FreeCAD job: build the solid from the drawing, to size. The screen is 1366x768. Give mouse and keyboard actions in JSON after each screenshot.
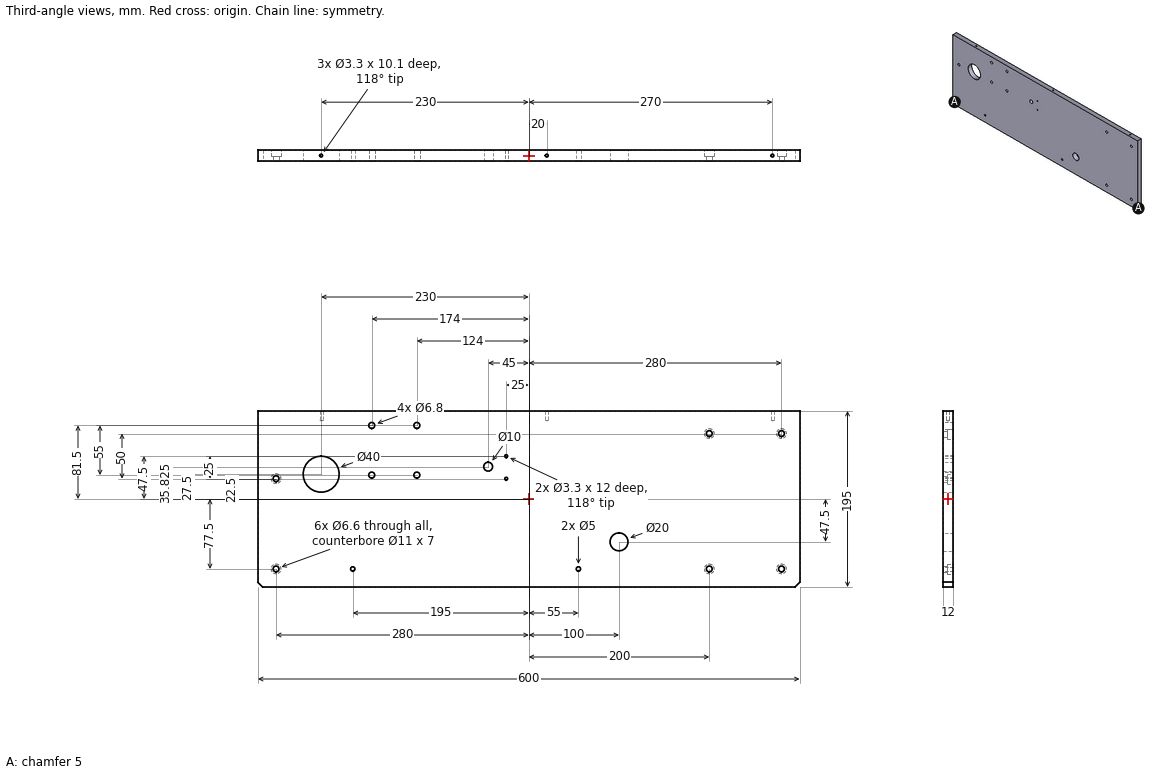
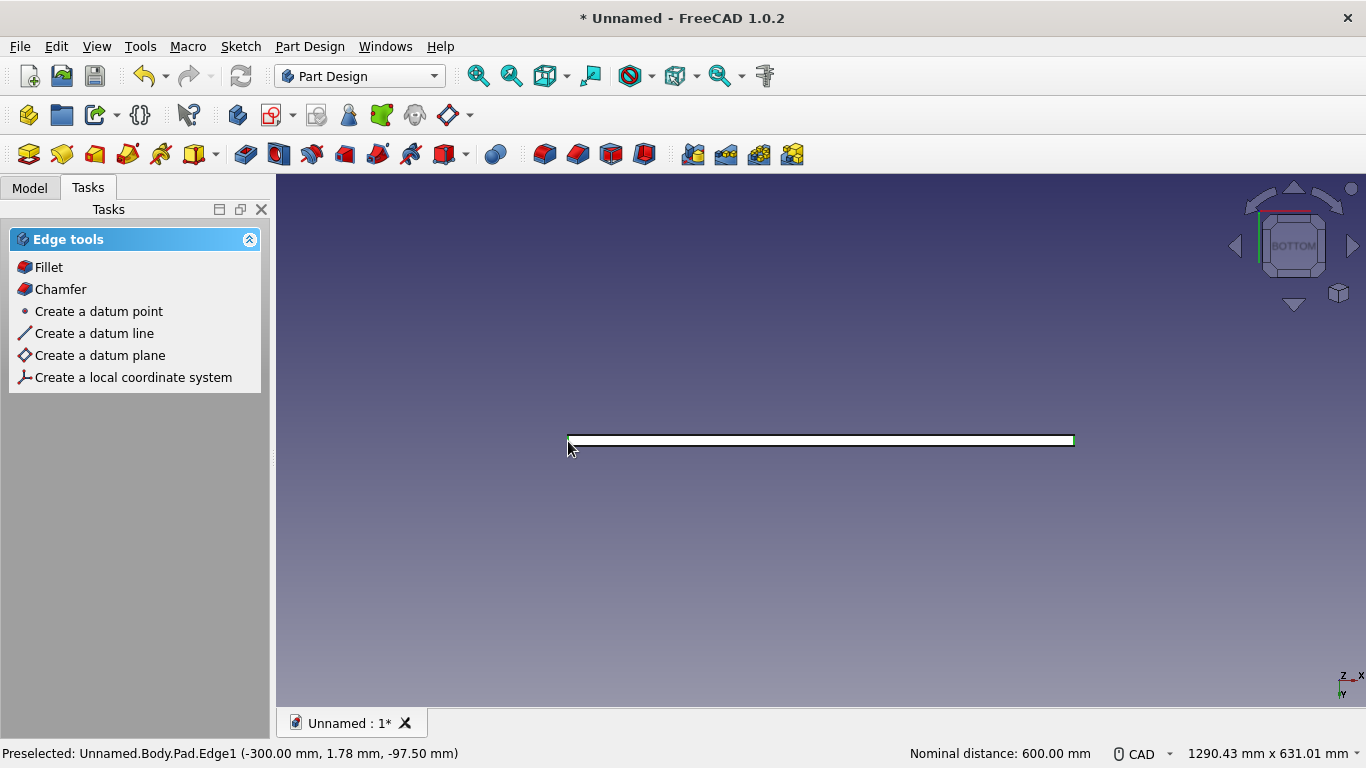
{"action": "left_click", "coordinate": [578, 154]}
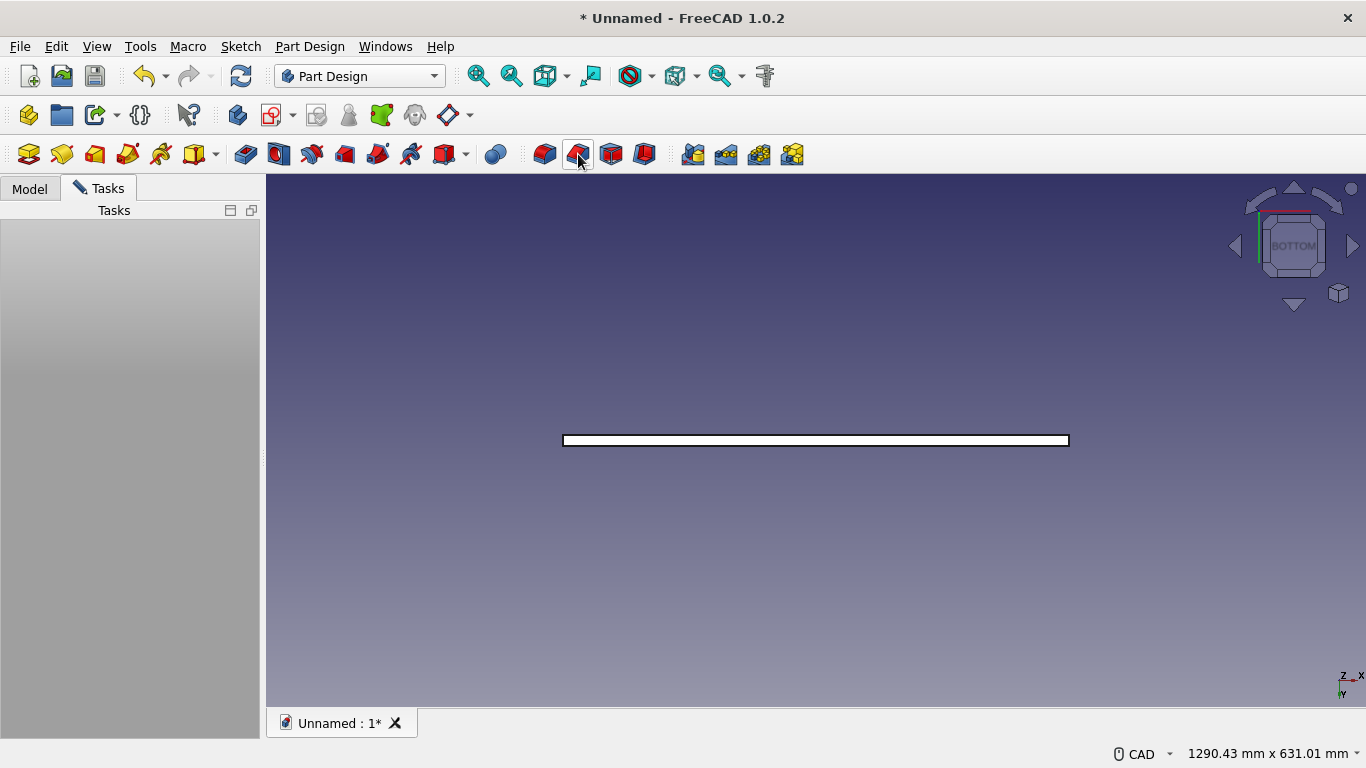
{"action": "type", "text": "5"}
{"action": "key", "text": "Tab"}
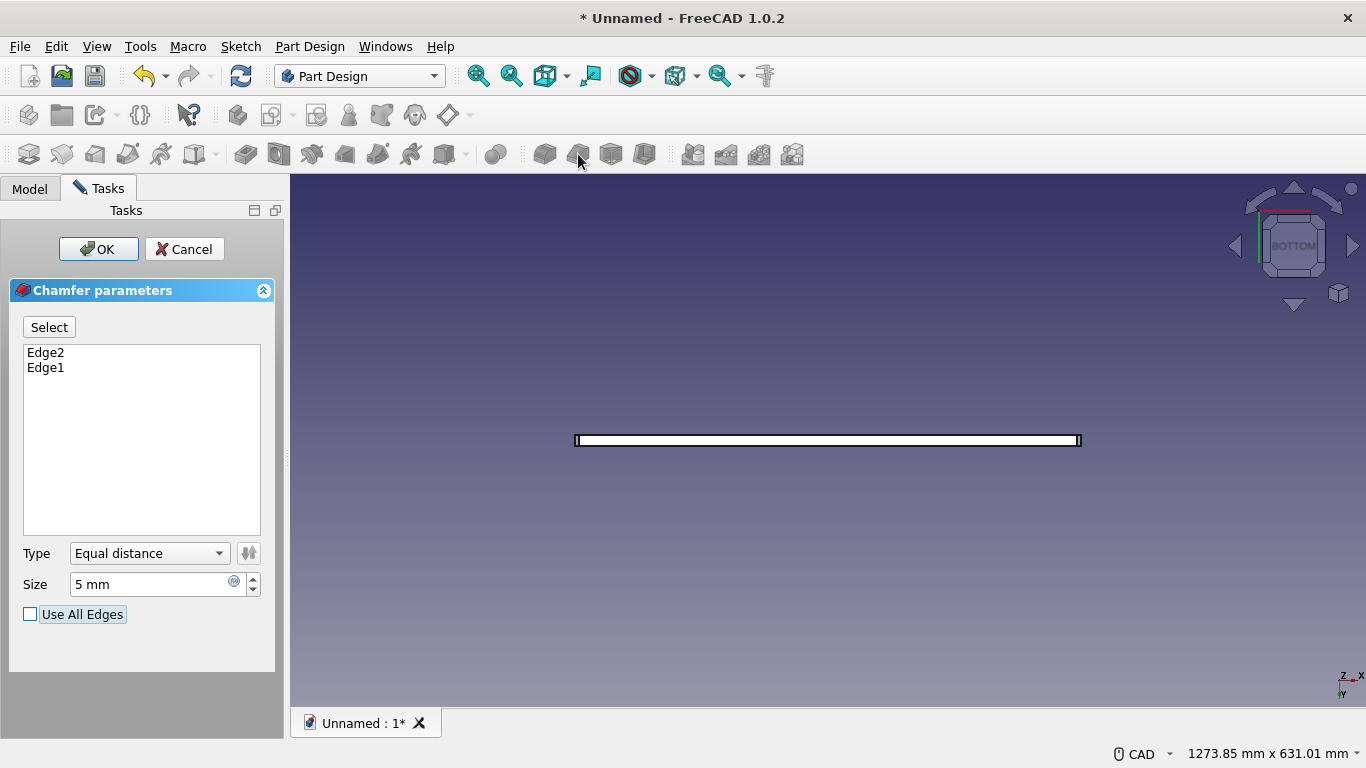
{"action": "left_click", "coordinate": [99, 249]}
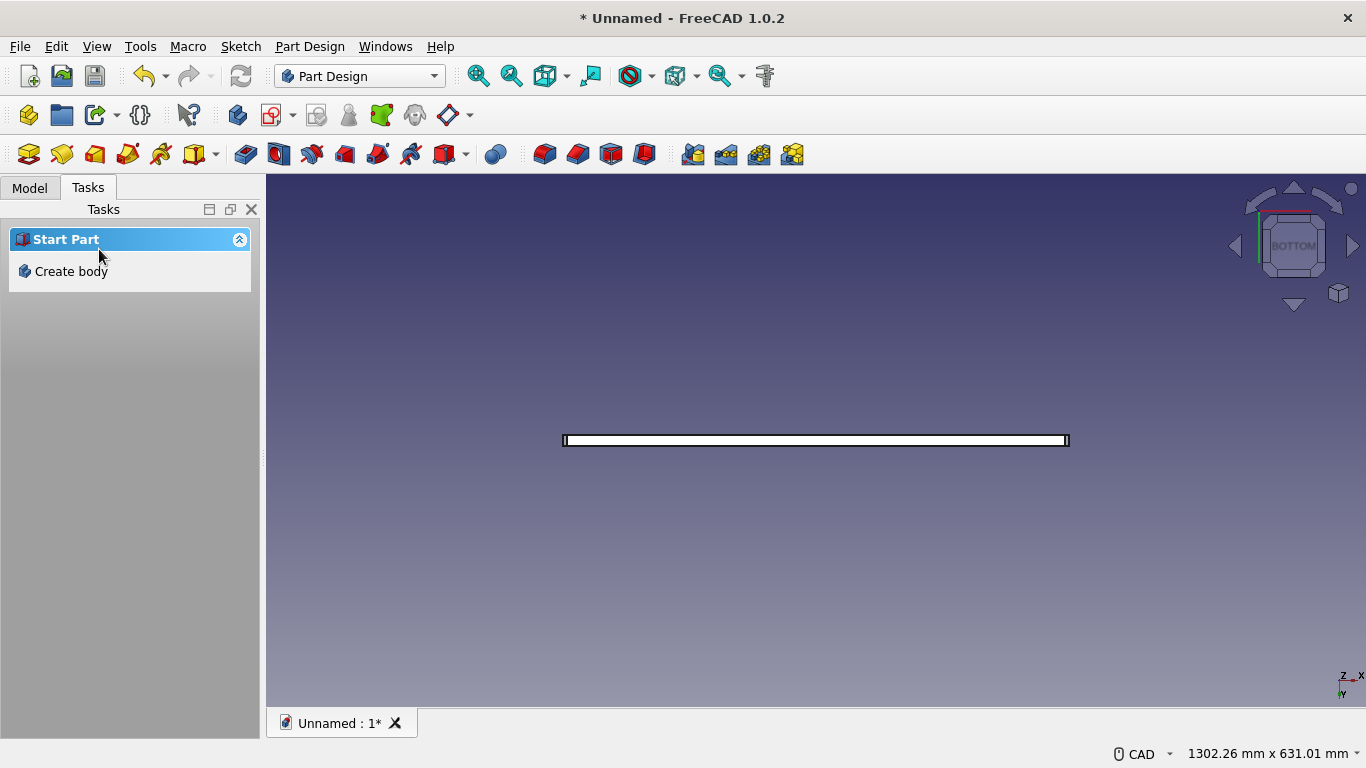
{"action": "key", "text": "4"}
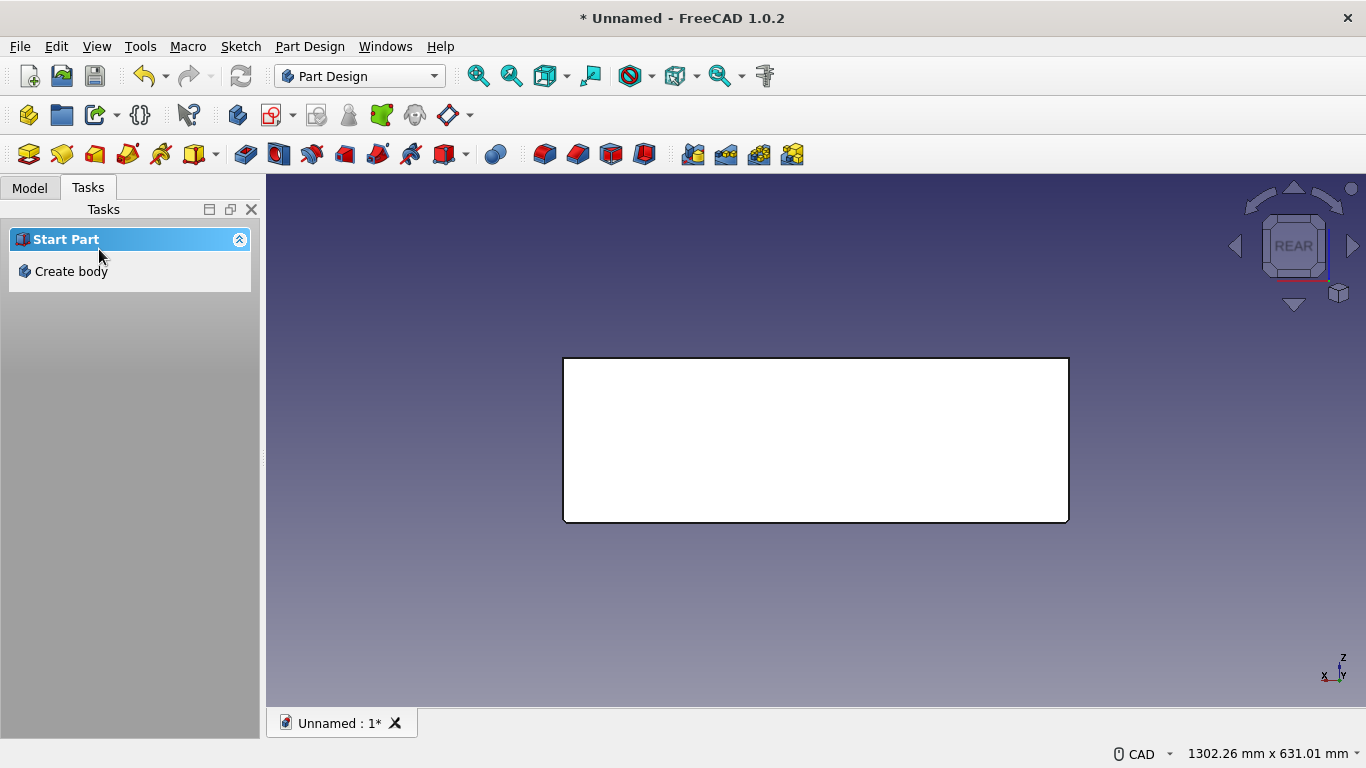
{"action": "left_click", "coordinate": [671, 439]}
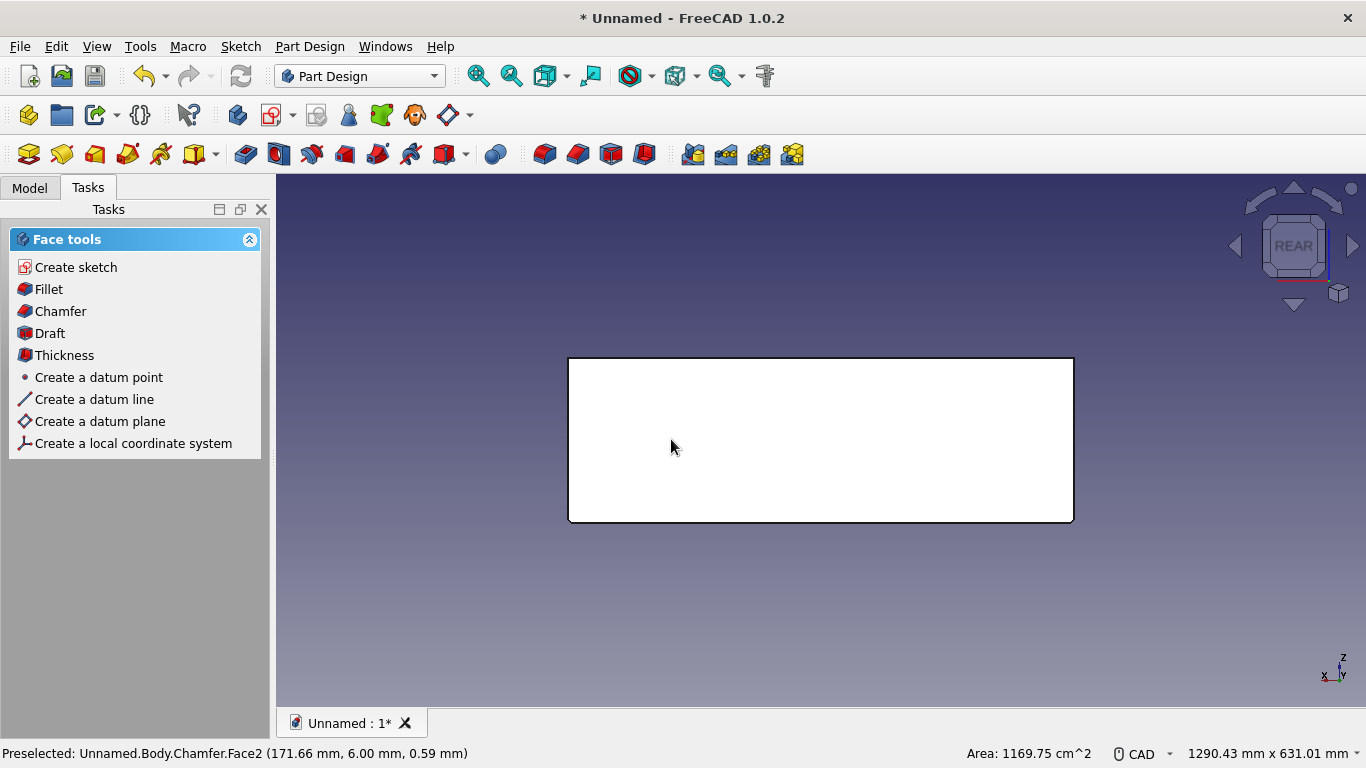
{"action": "left_click", "coordinate": [270, 116]}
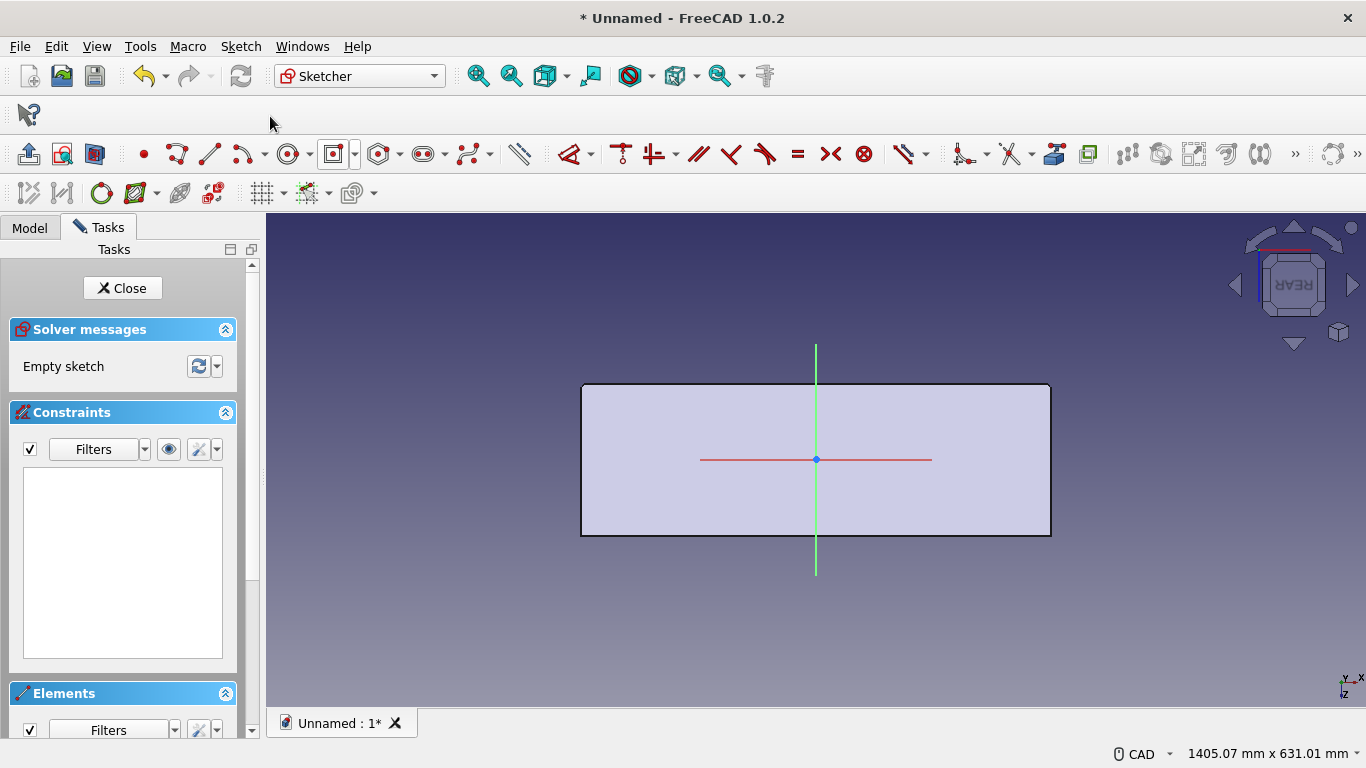
{"action": "scroll", "coordinate": [955, 454], "scroll_direction": "up", "scroll_amount": 2}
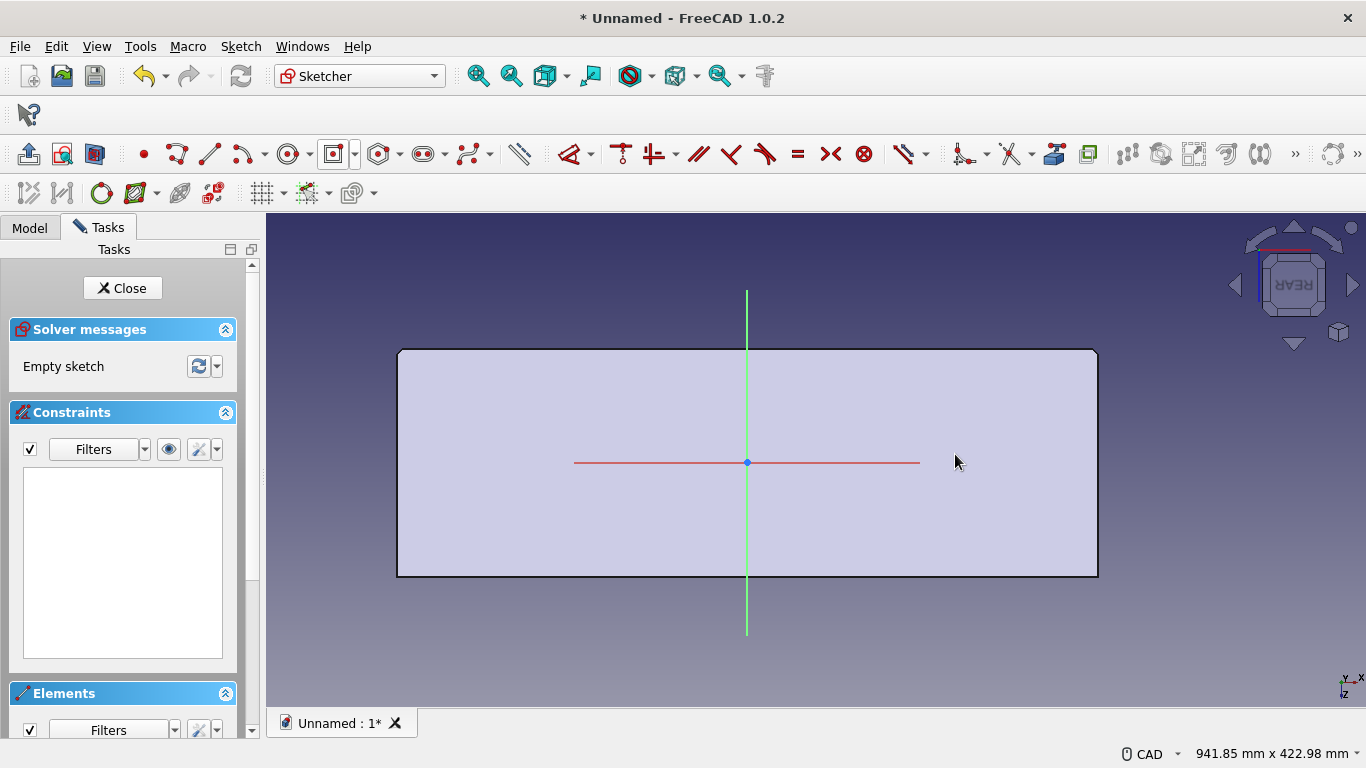
{"action": "left_click", "coordinate": [288, 154]}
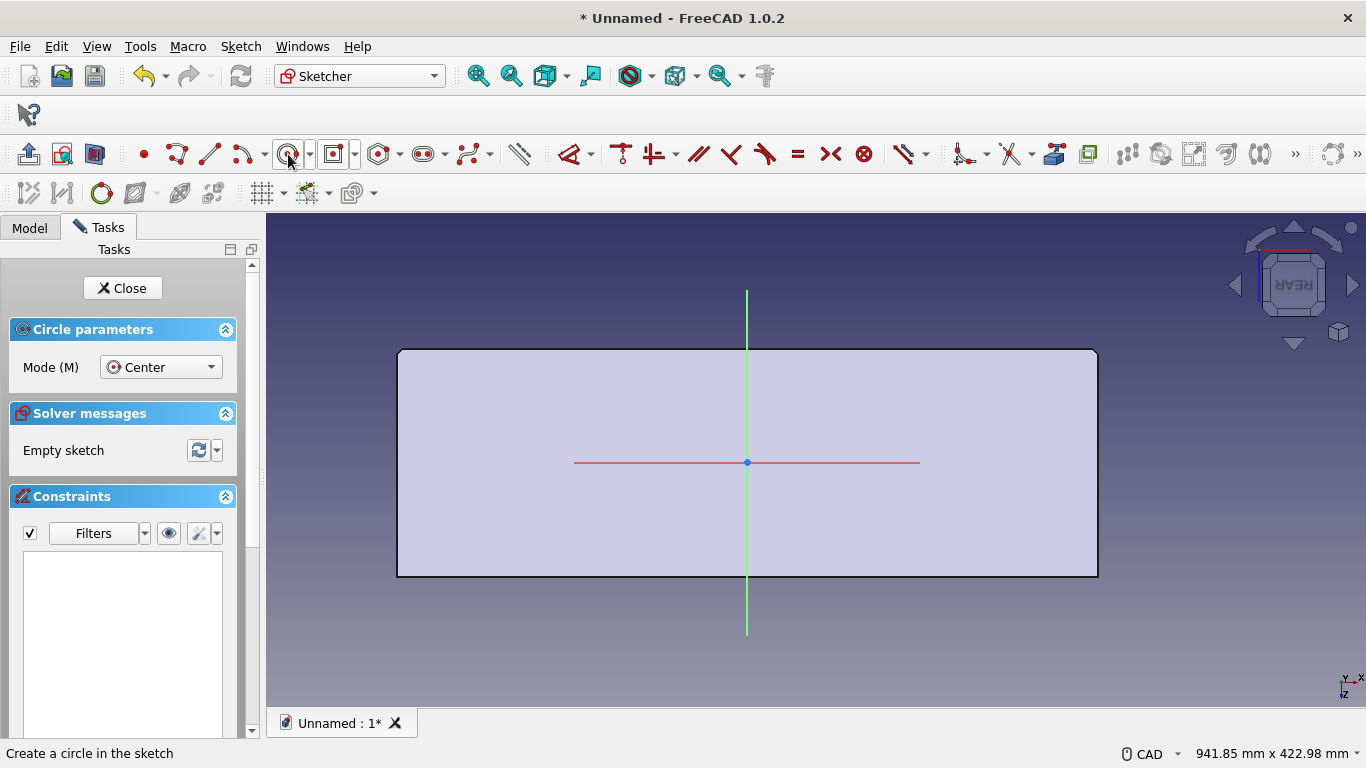
{"action": "scroll", "coordinate": [420, 372], "scroll_direction": "up", "scroll_amount": 9}